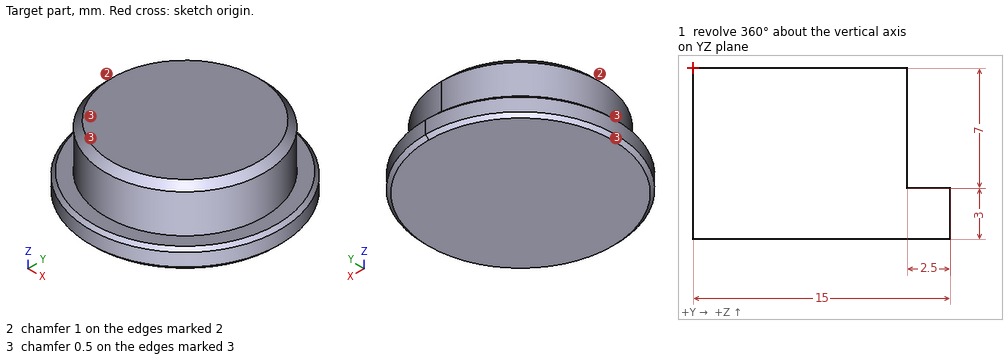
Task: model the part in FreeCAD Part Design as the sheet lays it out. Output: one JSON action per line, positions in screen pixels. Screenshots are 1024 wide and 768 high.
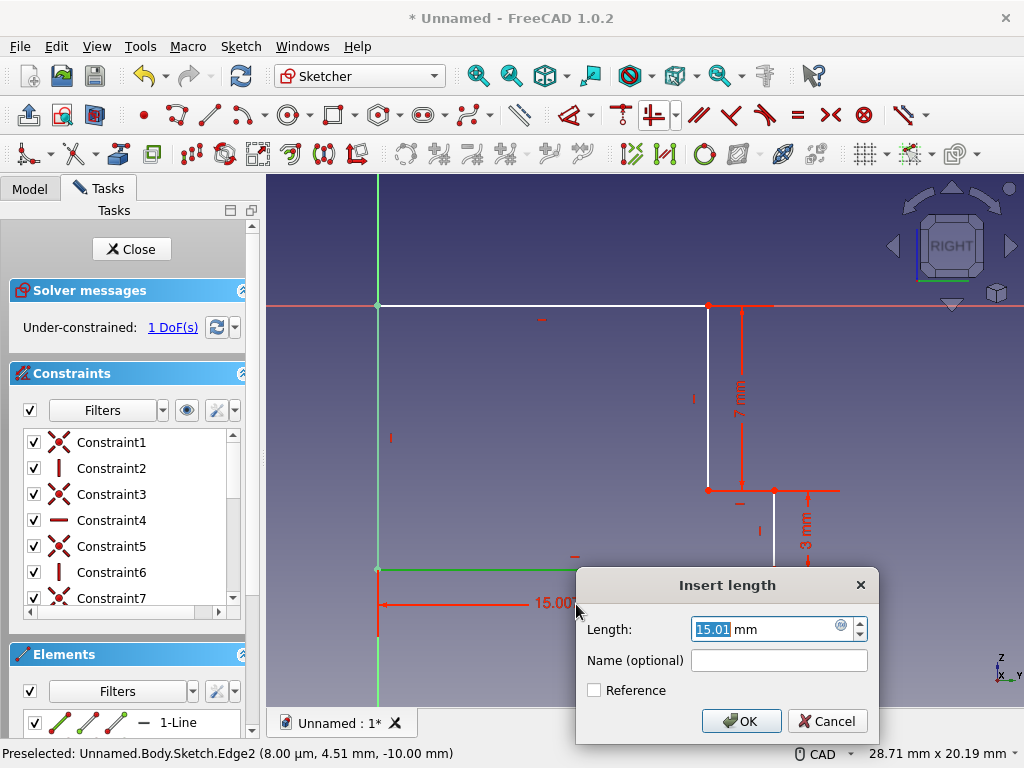
{"action": "type", "text": "15"}
{"action": "key", "text": "Return"}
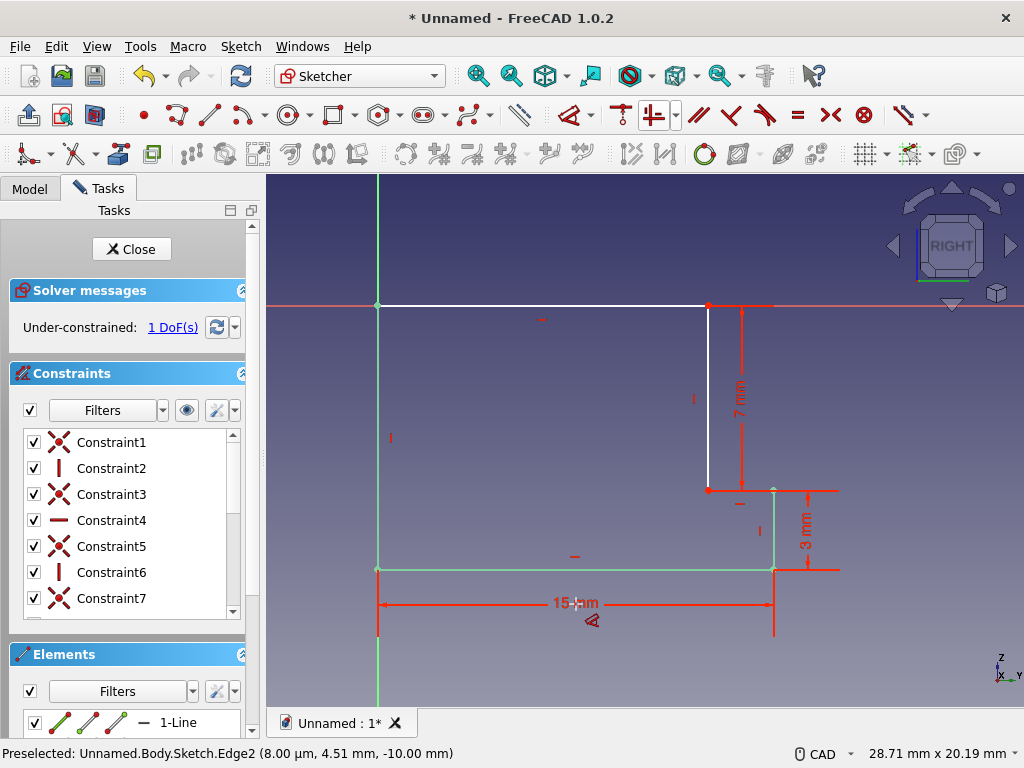
{"action": "left_click", "coordinate": [754, 491]}
{"action": "left_click", "coordinate": [726, 525]}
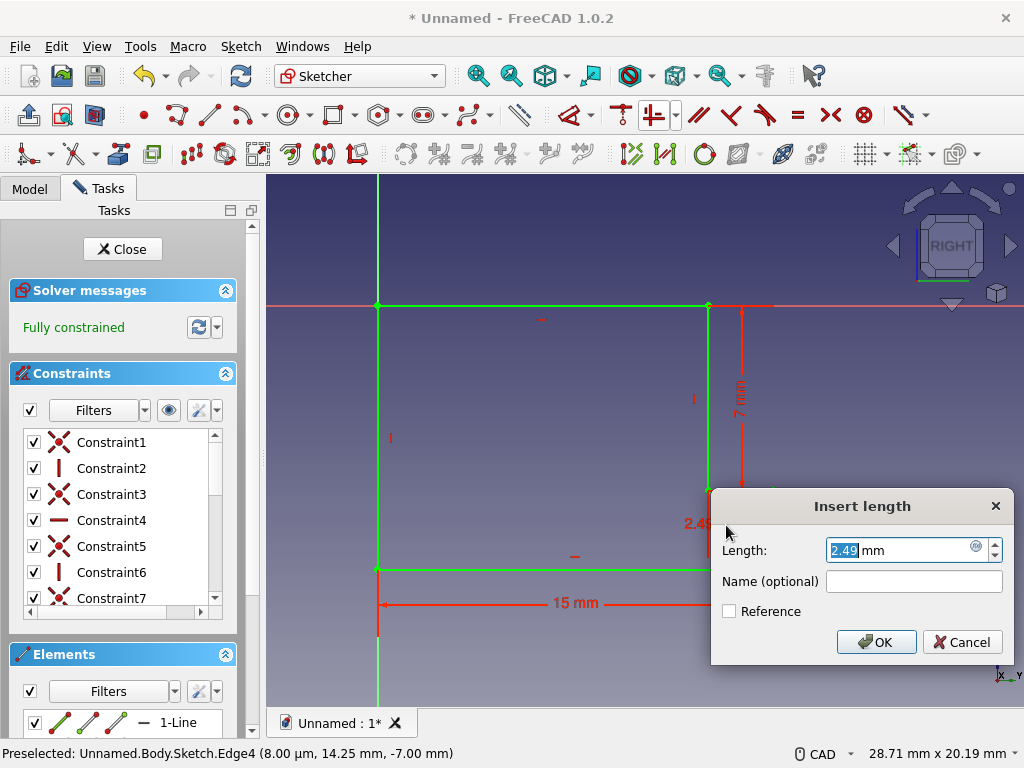
{"action": "type", "text": "2.5"}
{"action": "key", "text": "Return"}
{"action": "key", "text": "Escape"}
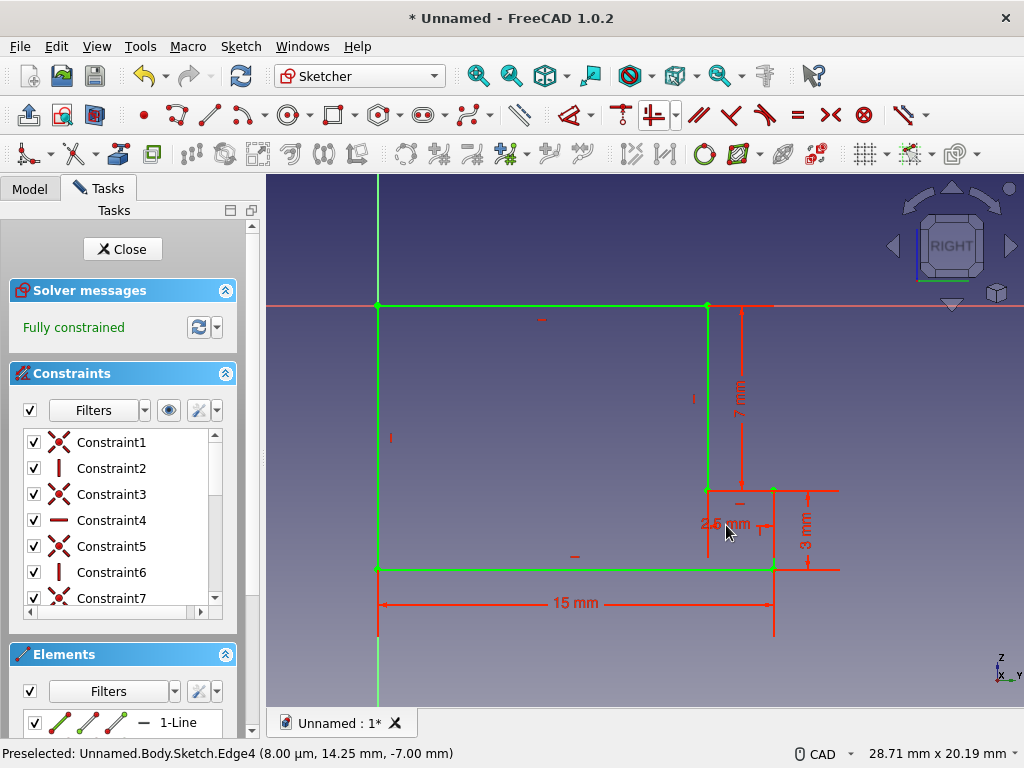
{"action": "left_click", "coordinate": [123, 249]}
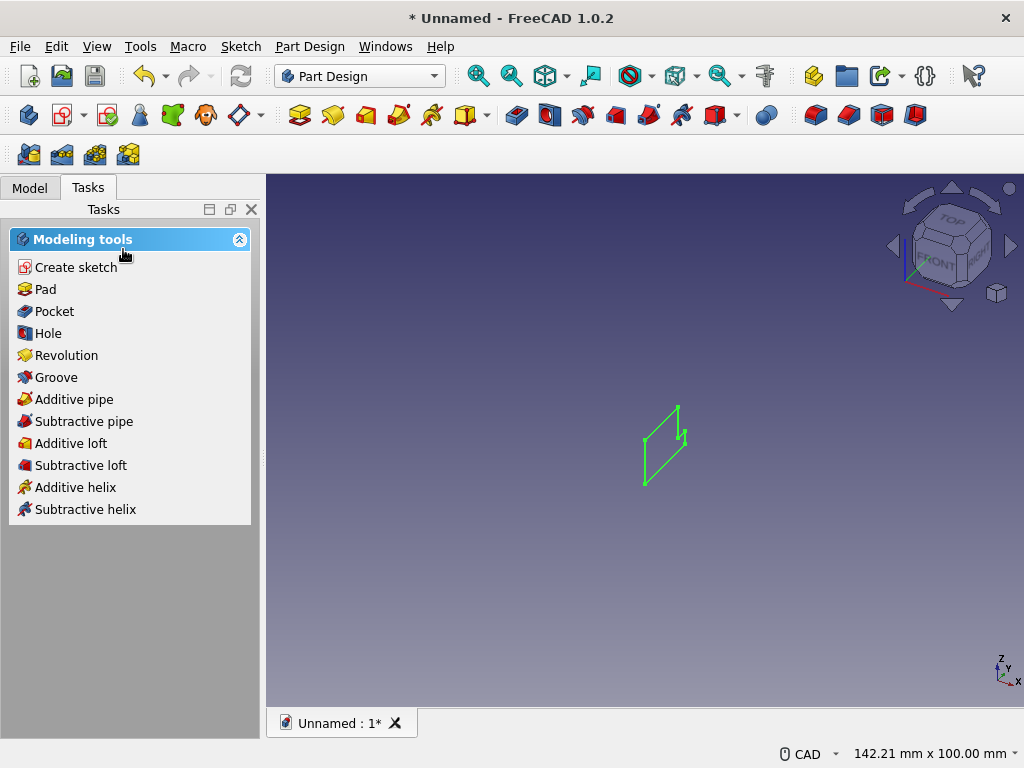
{"action": "left_click", "coordinate": [333, 116]}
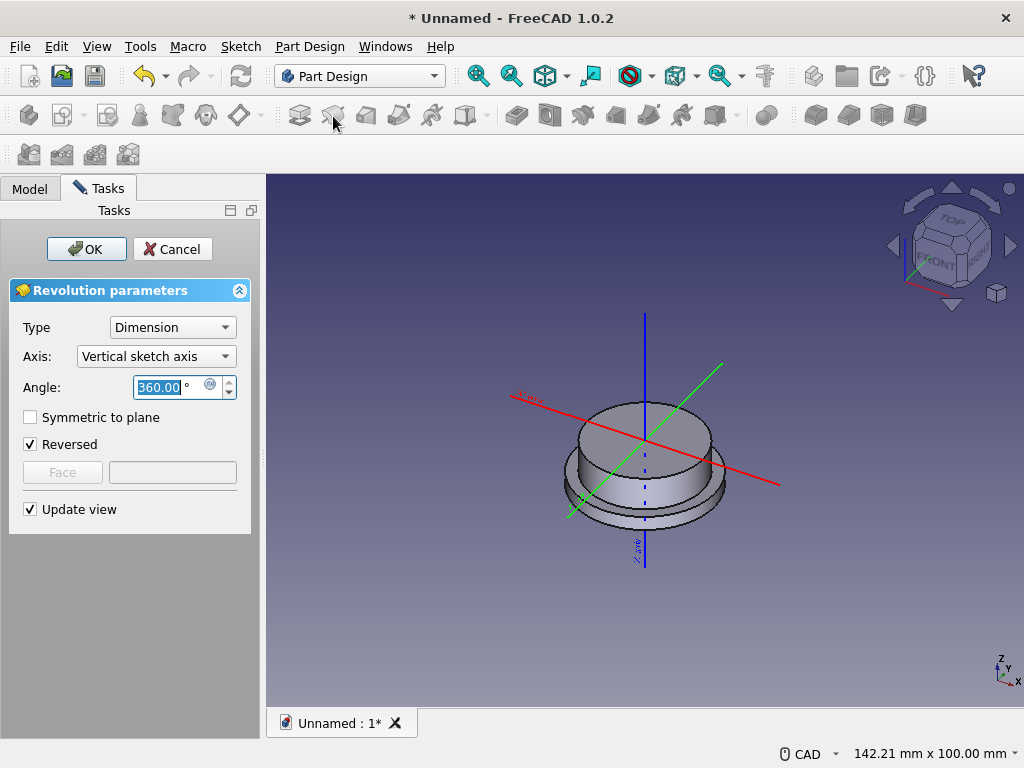
{"action": "left_click", "coordinate": [87, 249]}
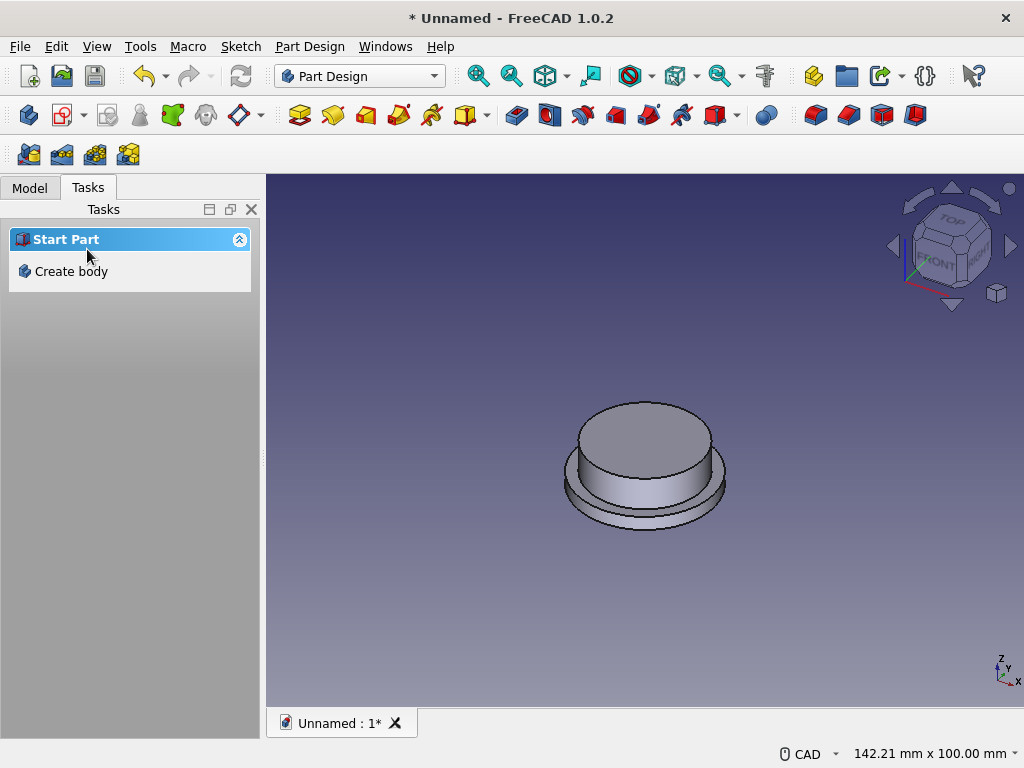
{"action": "key", "text": "v f"}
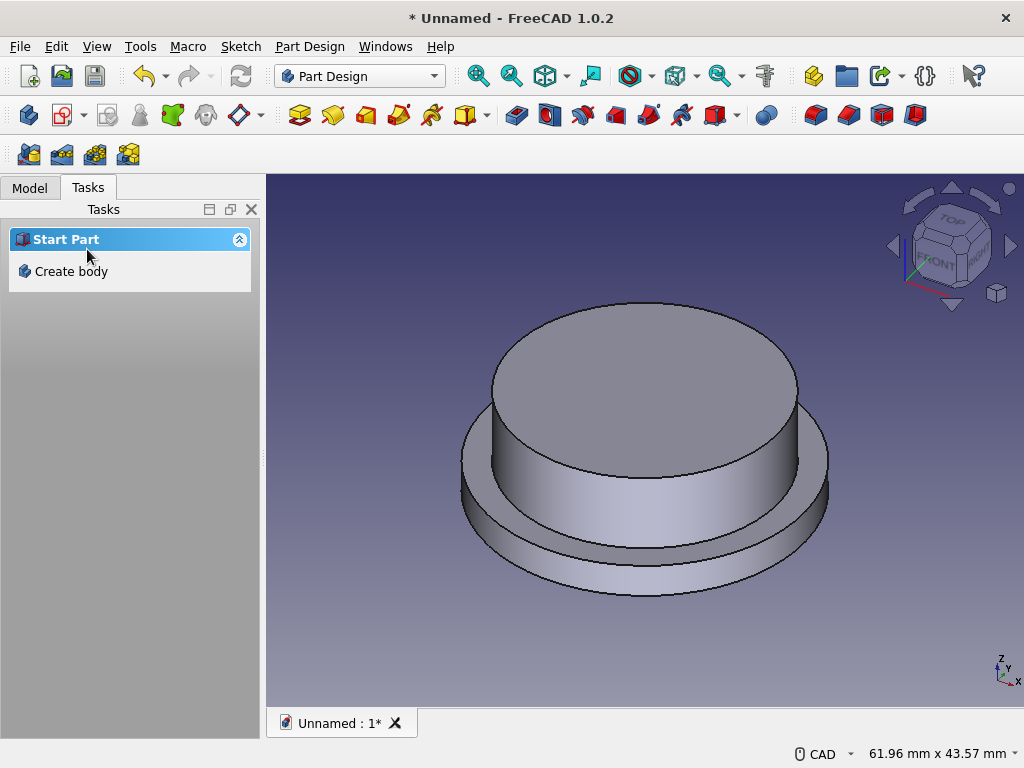
{"action": "left_click", "coordinate": [568, 465]}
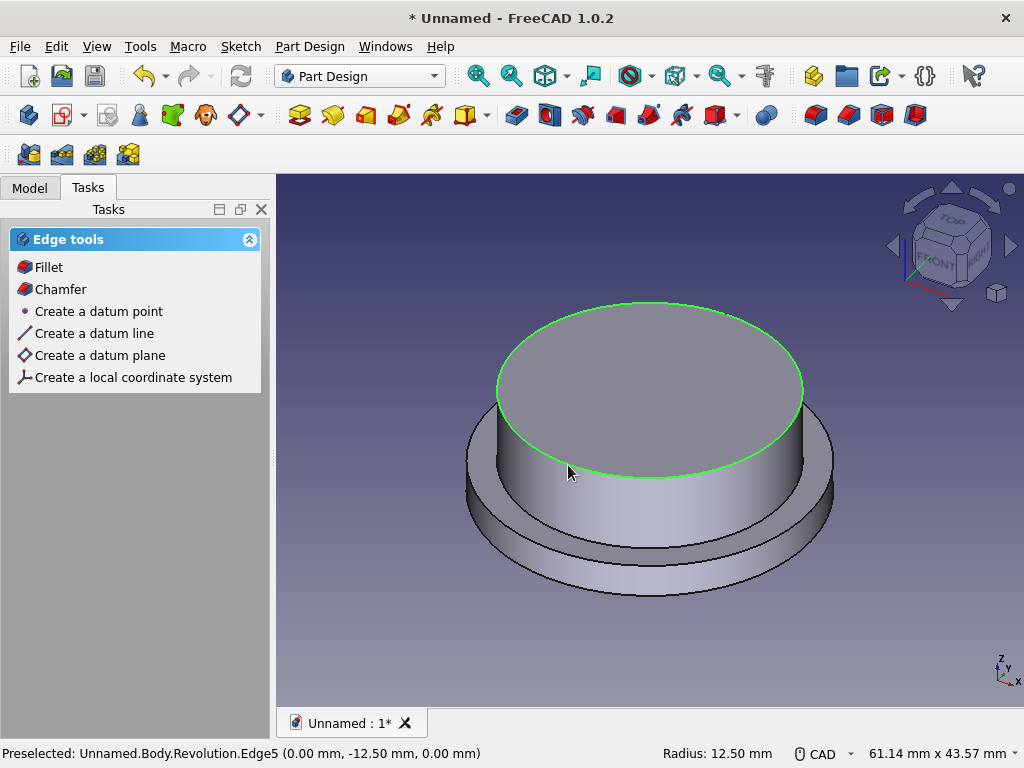
{"action": "left_click", "coordinate": [849, 116]}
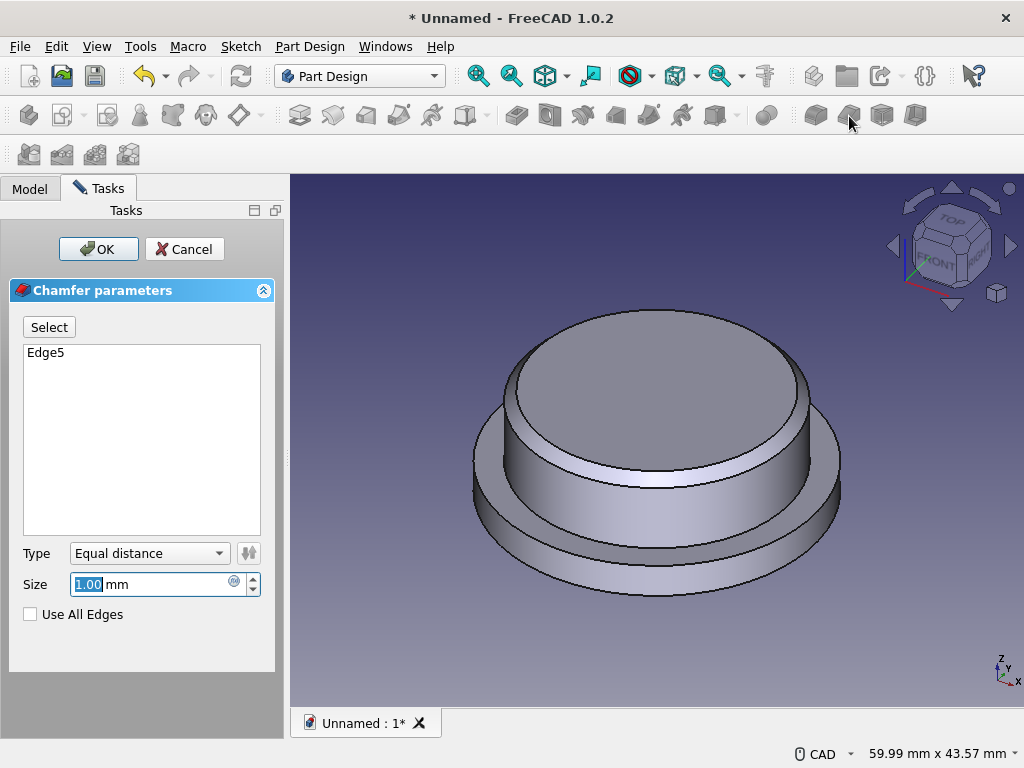
{"action": "type", "text": "1"}
{"action": "key", "text": "Tab"}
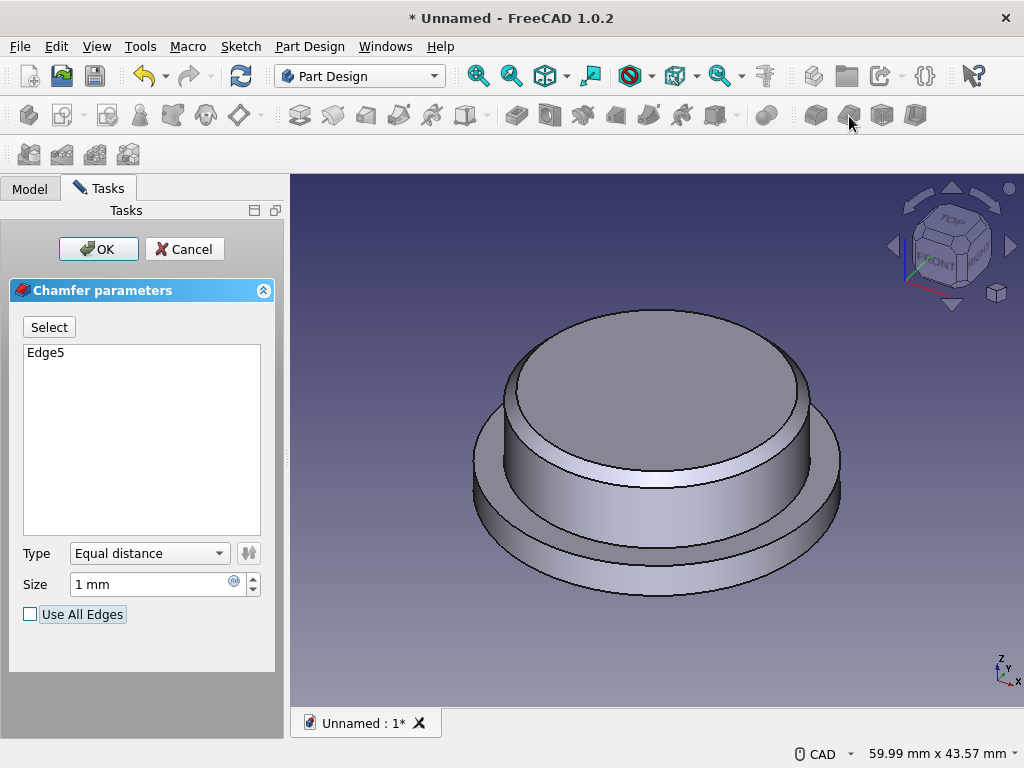
{"action": "left_click", "coordinate": [99, 249]}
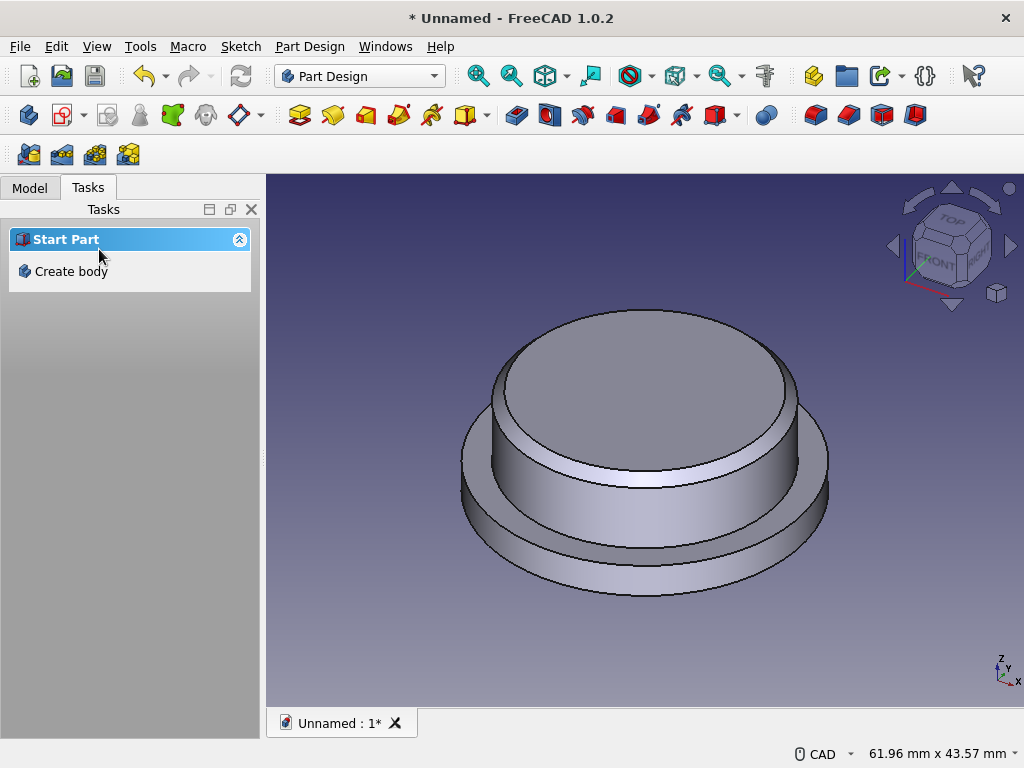
{"action": "left_click", "coordinate": [553, 551]}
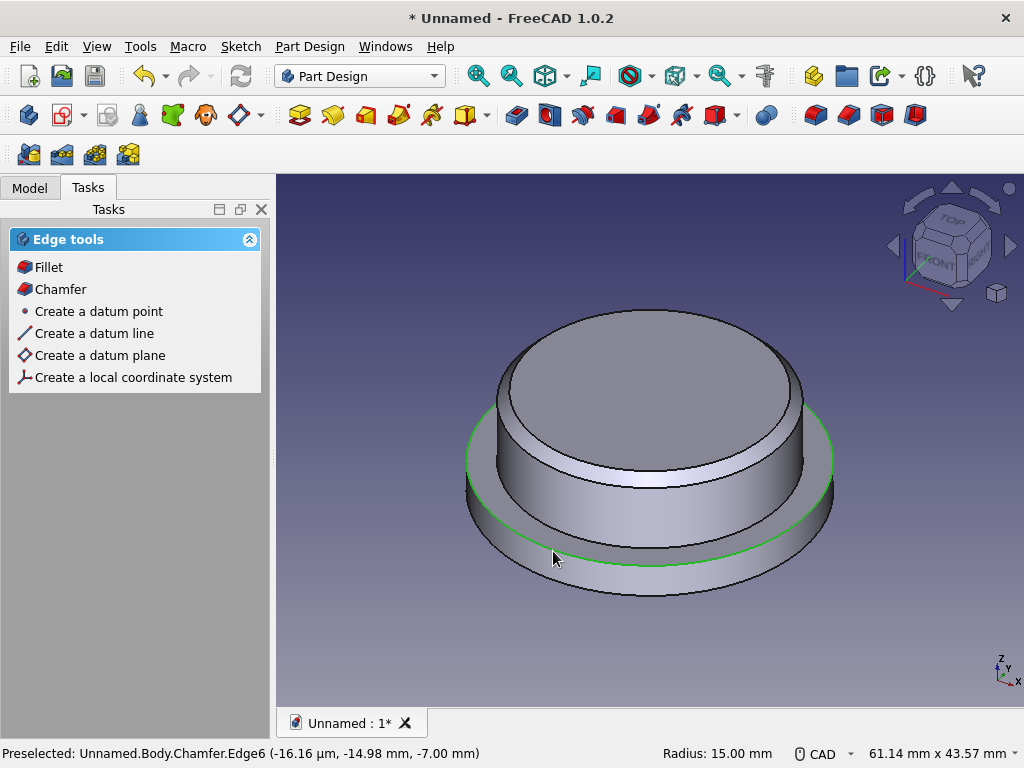
{"action": "key", "text": "0"}